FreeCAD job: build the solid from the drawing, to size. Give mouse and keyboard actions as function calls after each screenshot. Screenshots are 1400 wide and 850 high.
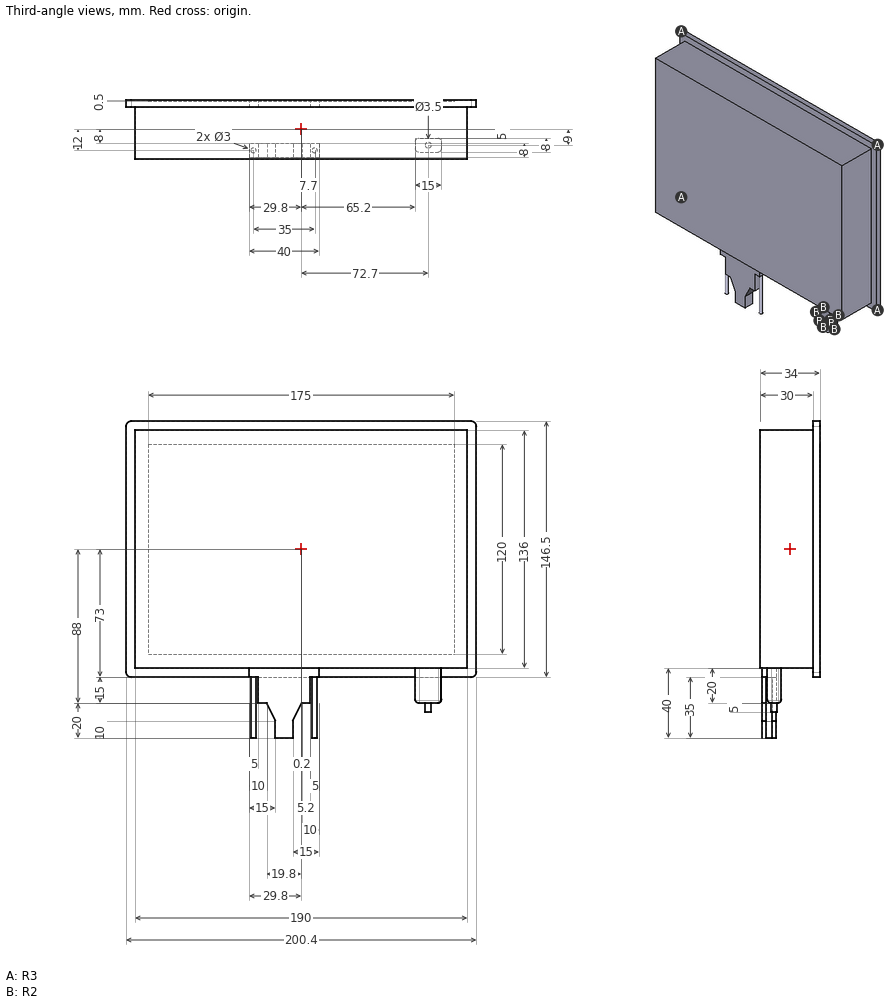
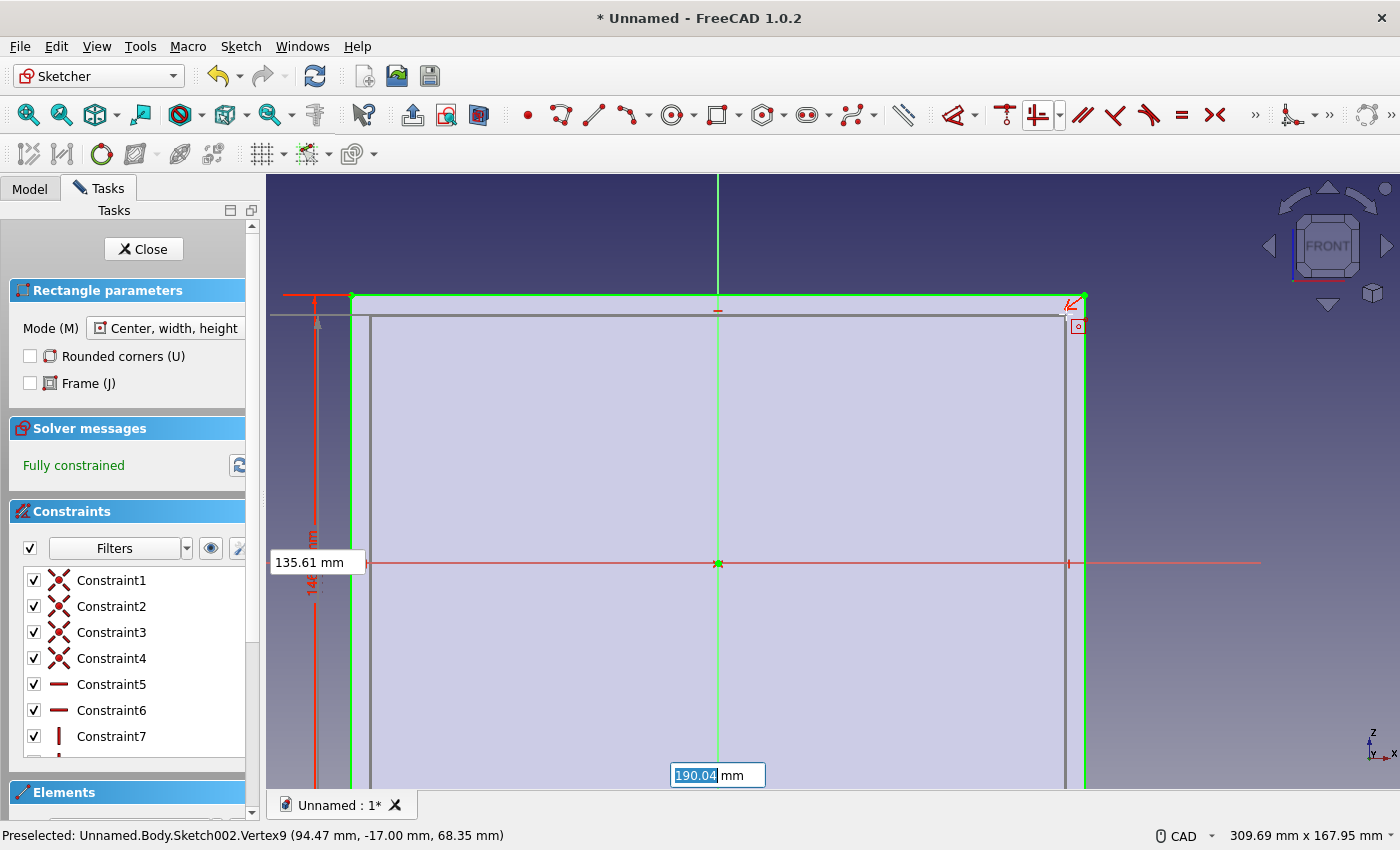
text(190)
key(Tab)
text(136)
key(Return)
key(Escape)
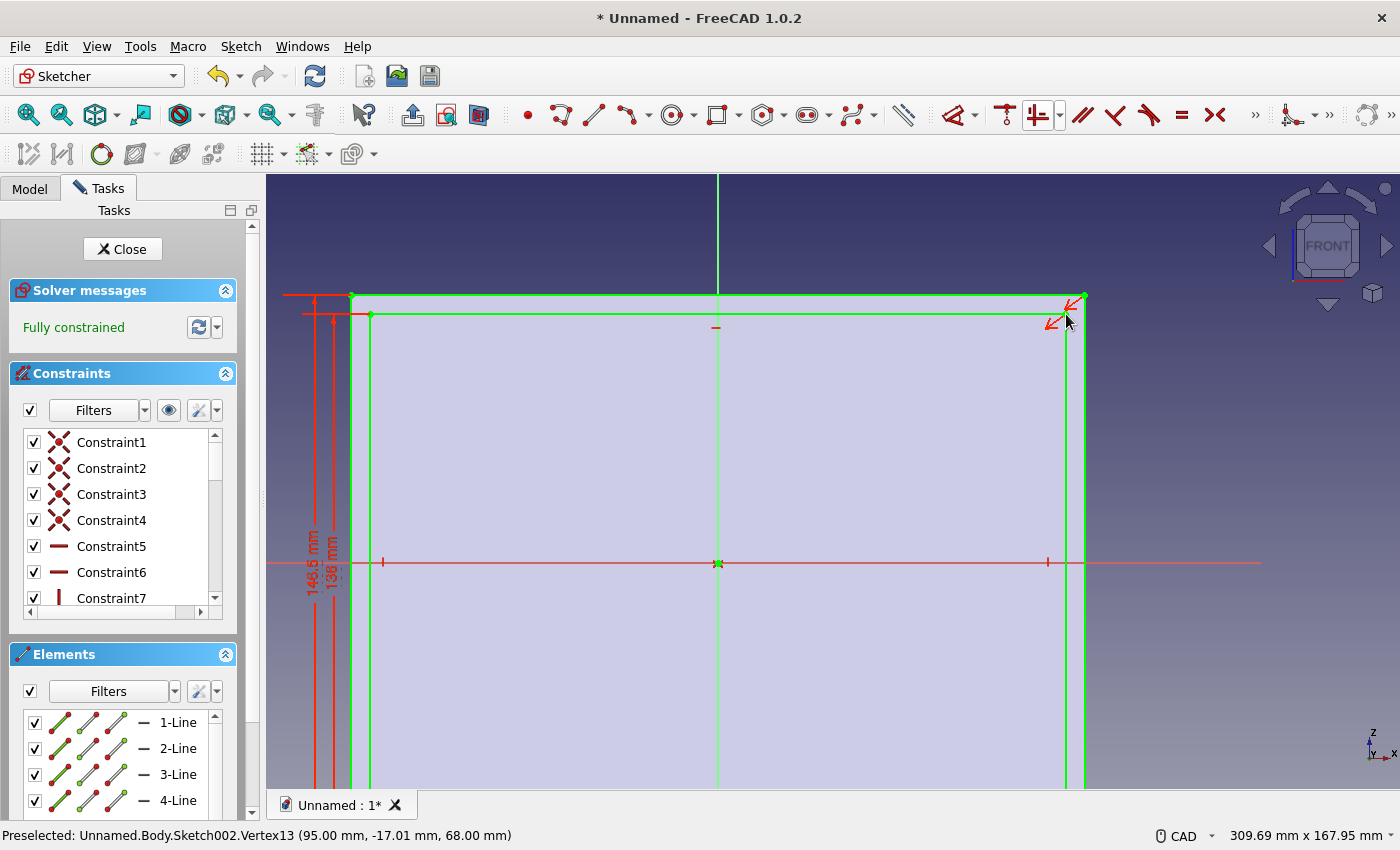
click(123, 249)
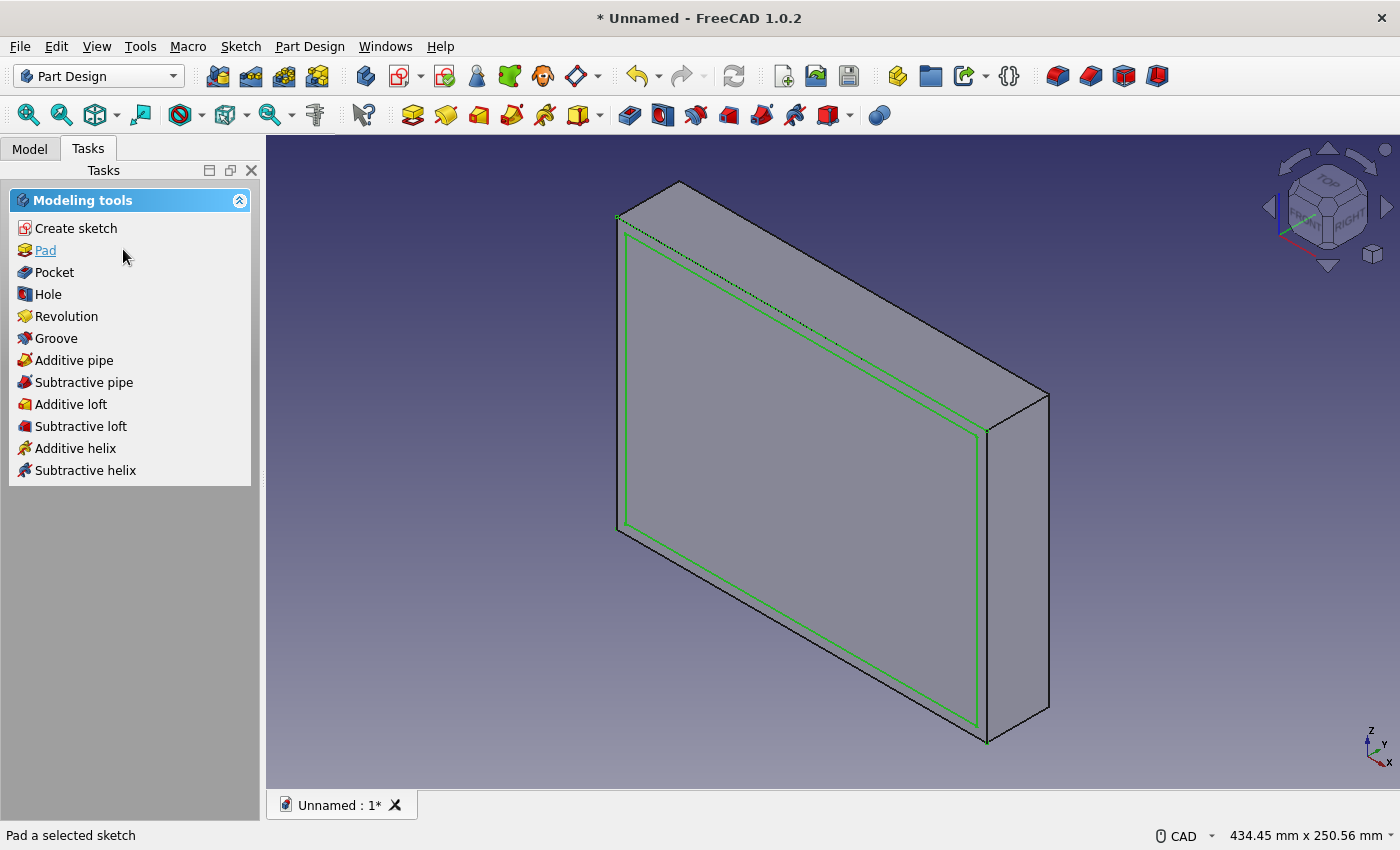
click(630, 116)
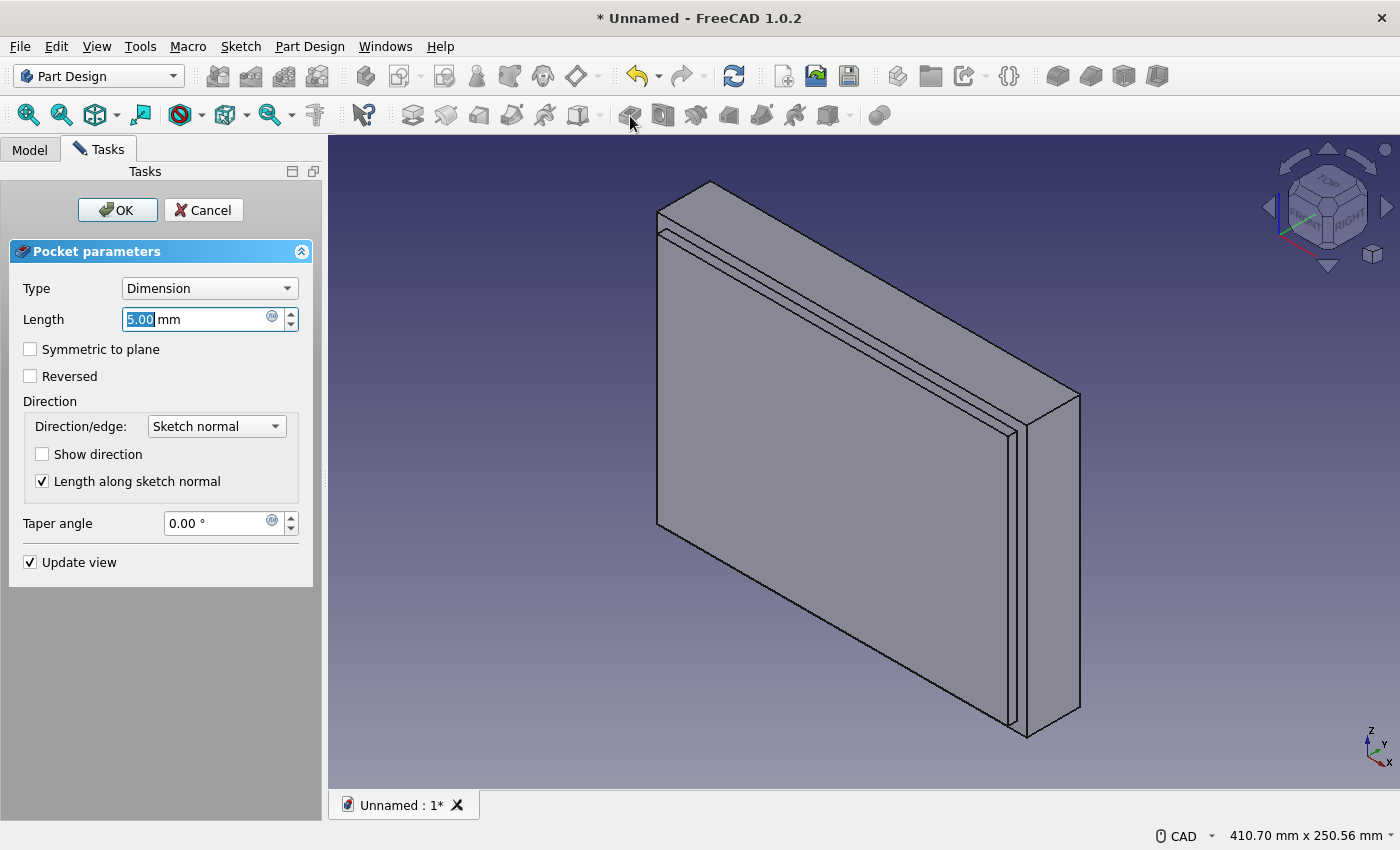
text(30)
key(Tab)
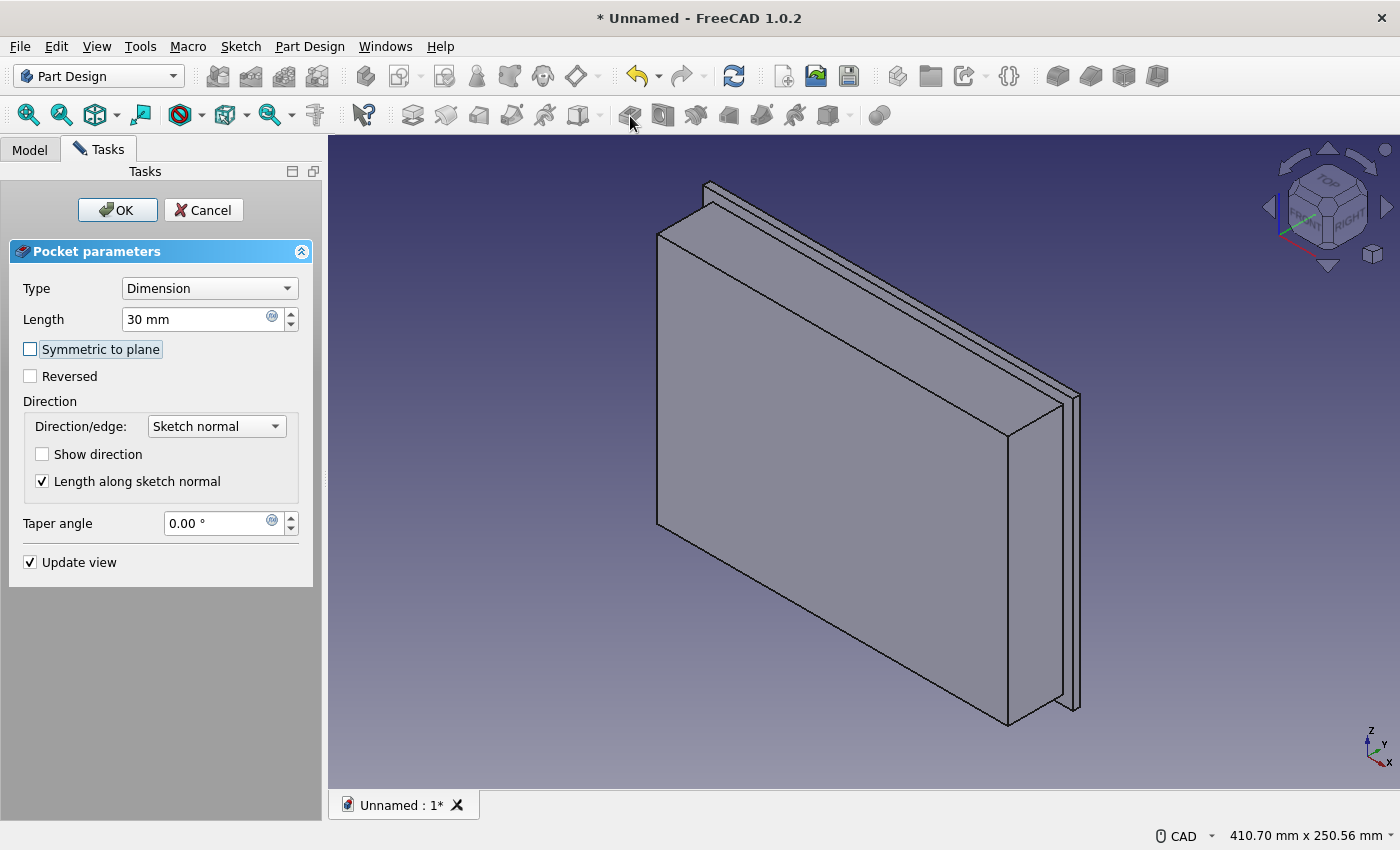
click(118, 210)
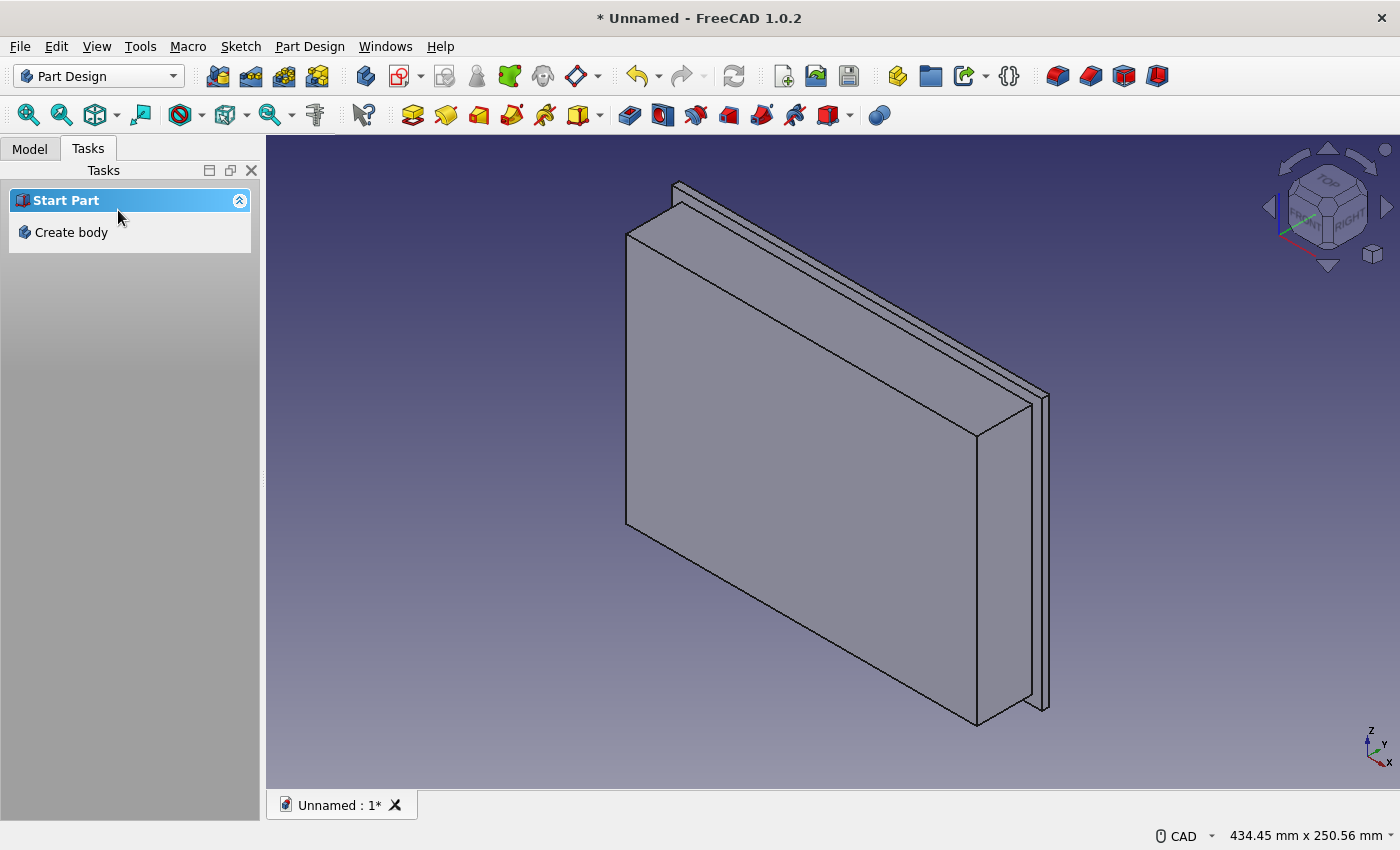
scroll(676, 494, up, 7)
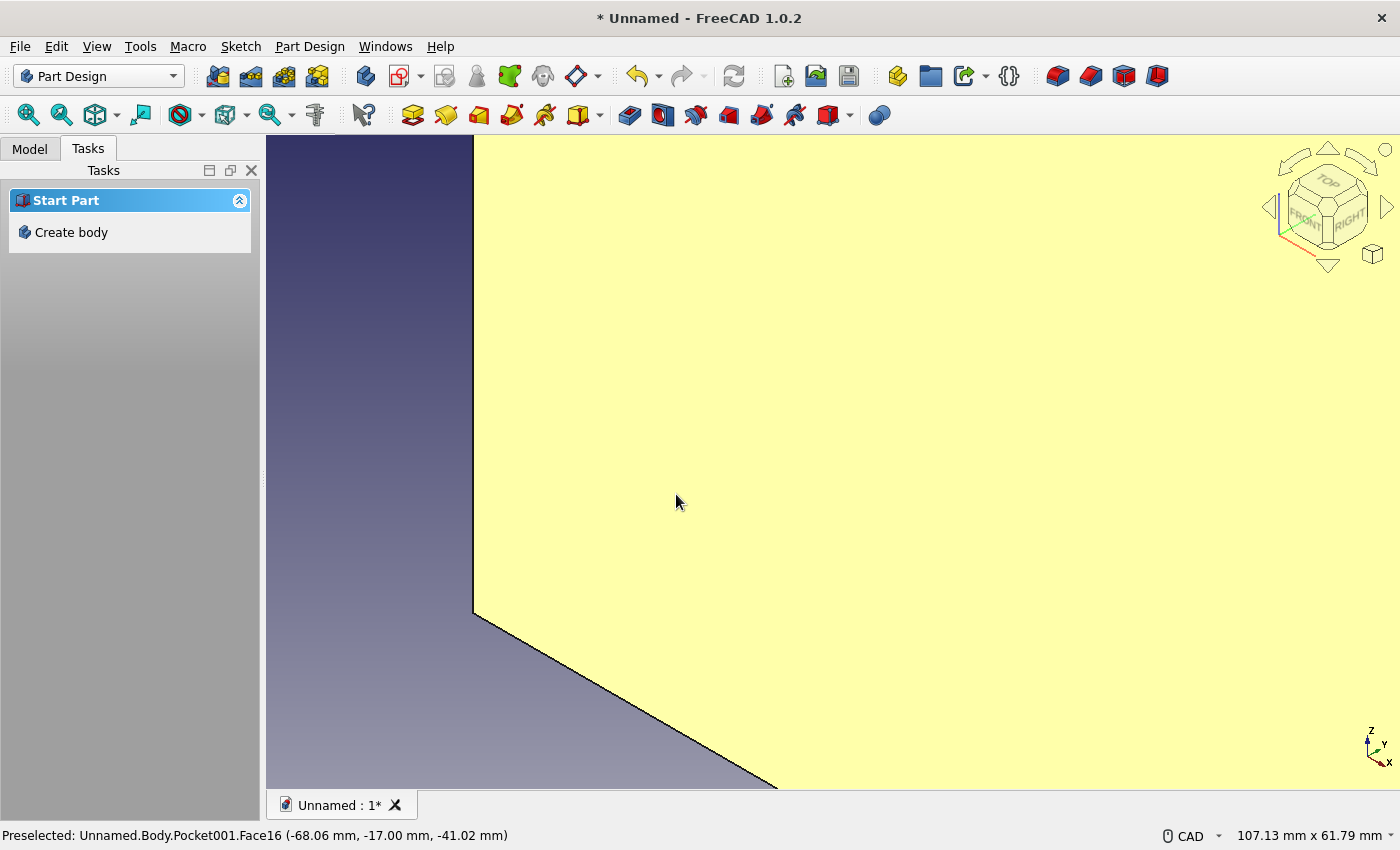
click(29, 116)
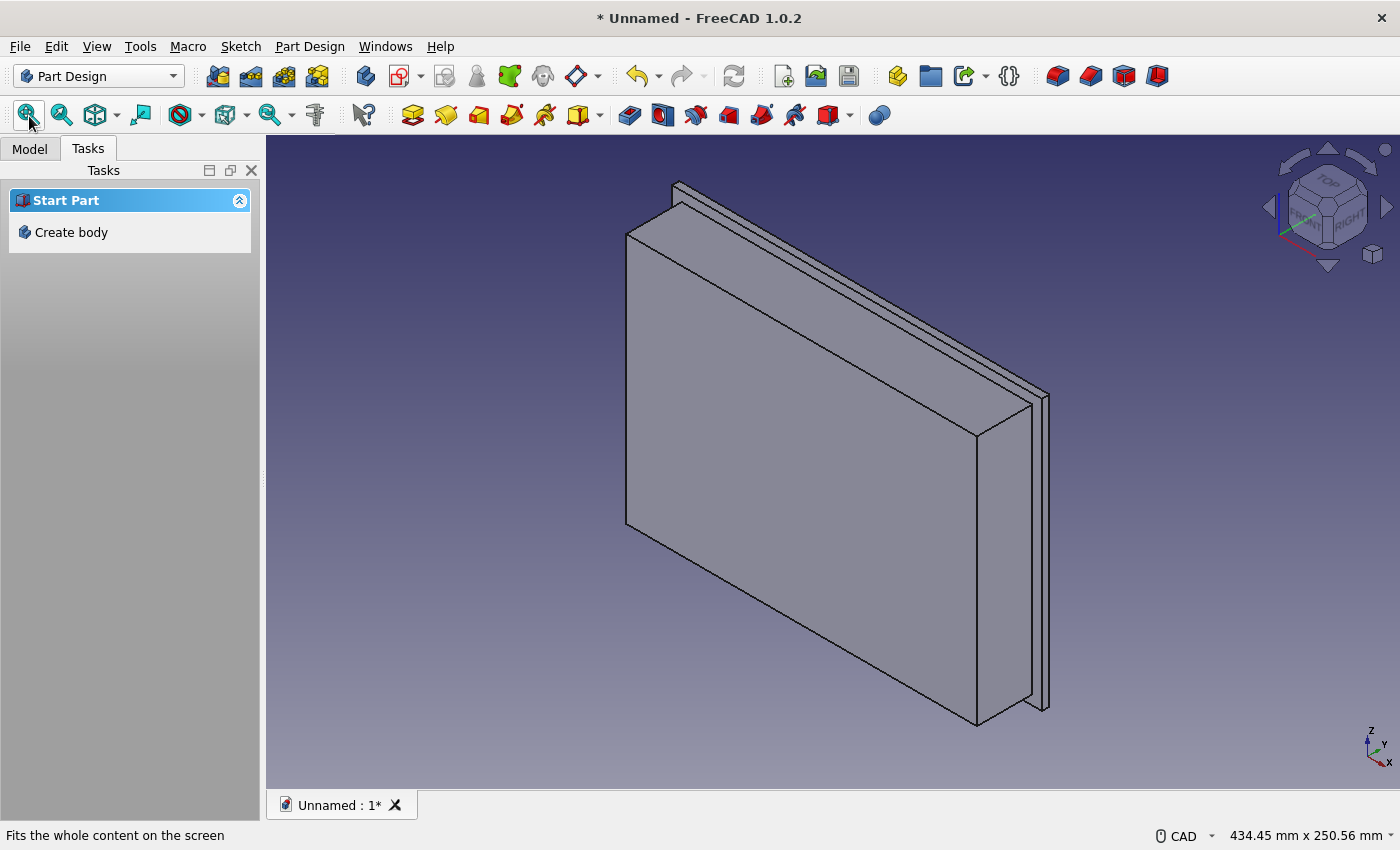
key(2)